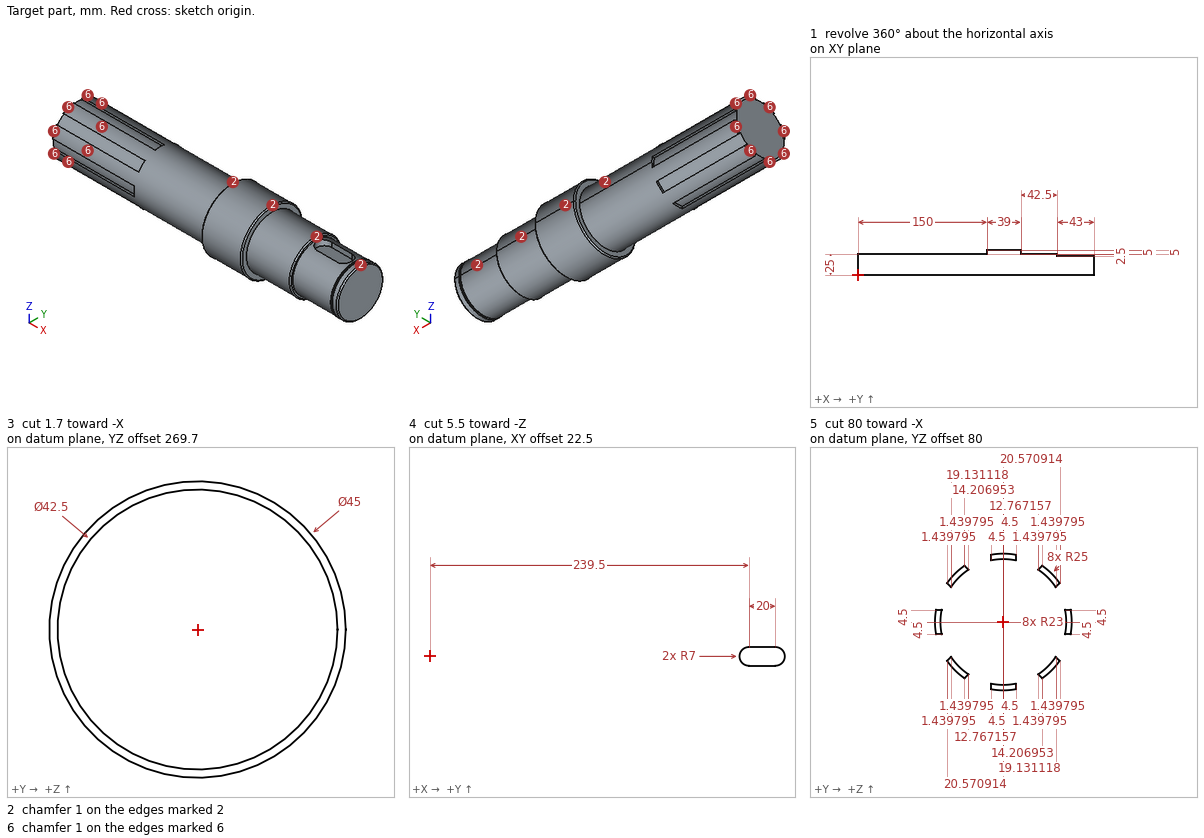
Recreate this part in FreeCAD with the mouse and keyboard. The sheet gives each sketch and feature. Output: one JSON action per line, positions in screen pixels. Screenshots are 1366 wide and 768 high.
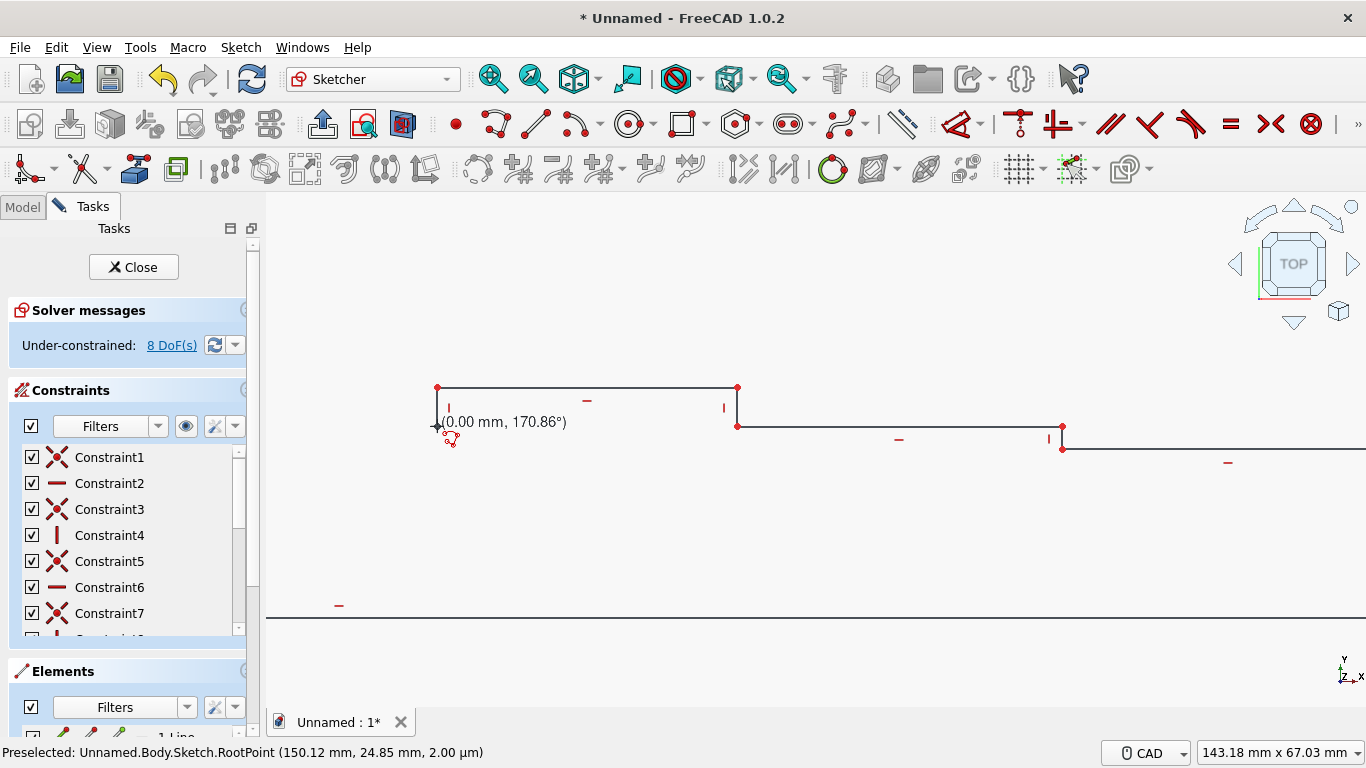
{"action": "scroll", "coordinate": [924, 427], "scroll_direction": "down", "scroll_amount": 6}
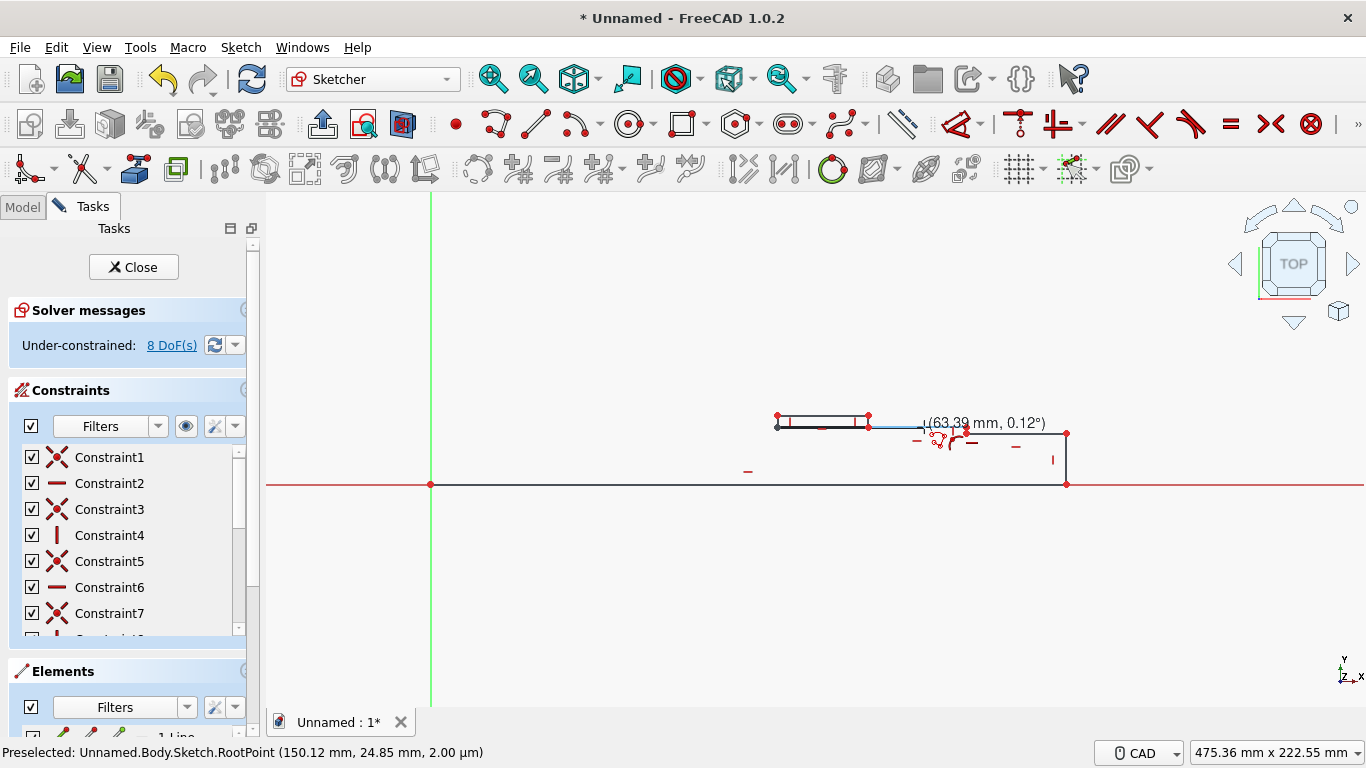
{"action": "left_click", "coordinate": [440, 427]}
{"action": "left_click", "coordinate": [431, 485]}
{"action": "key", "text": "Escape"}
{"action": "key", "text": "Escape"}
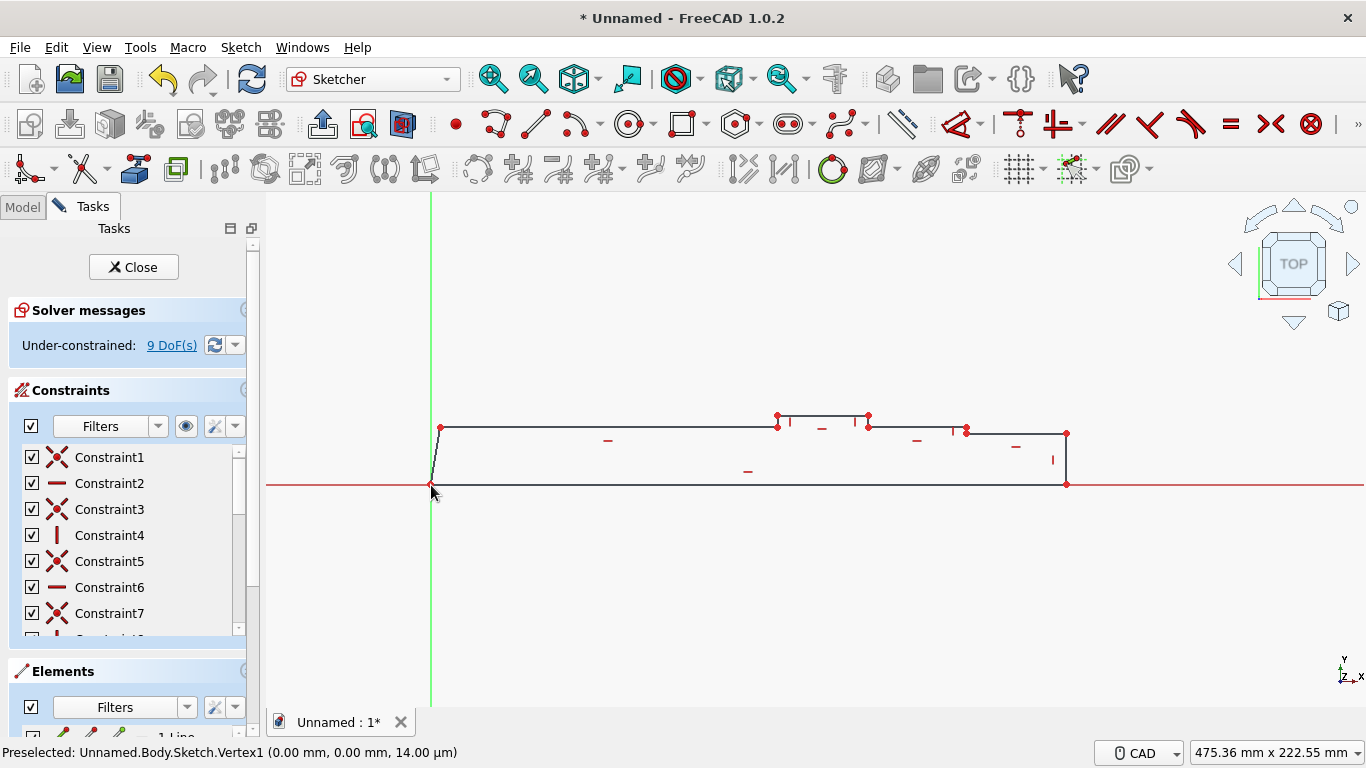
{"action": "left_click", "coordinate": [433, 468]}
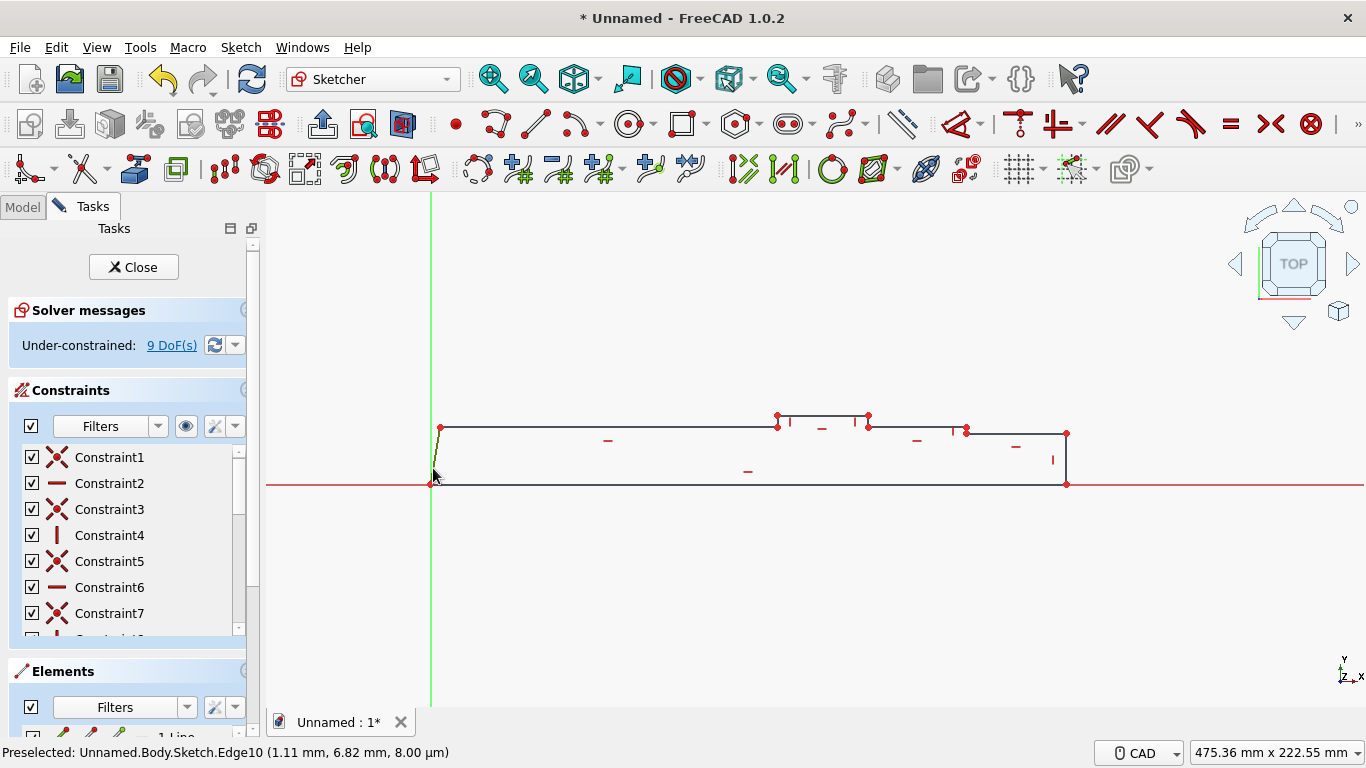
{"action": "key", "text": "v"}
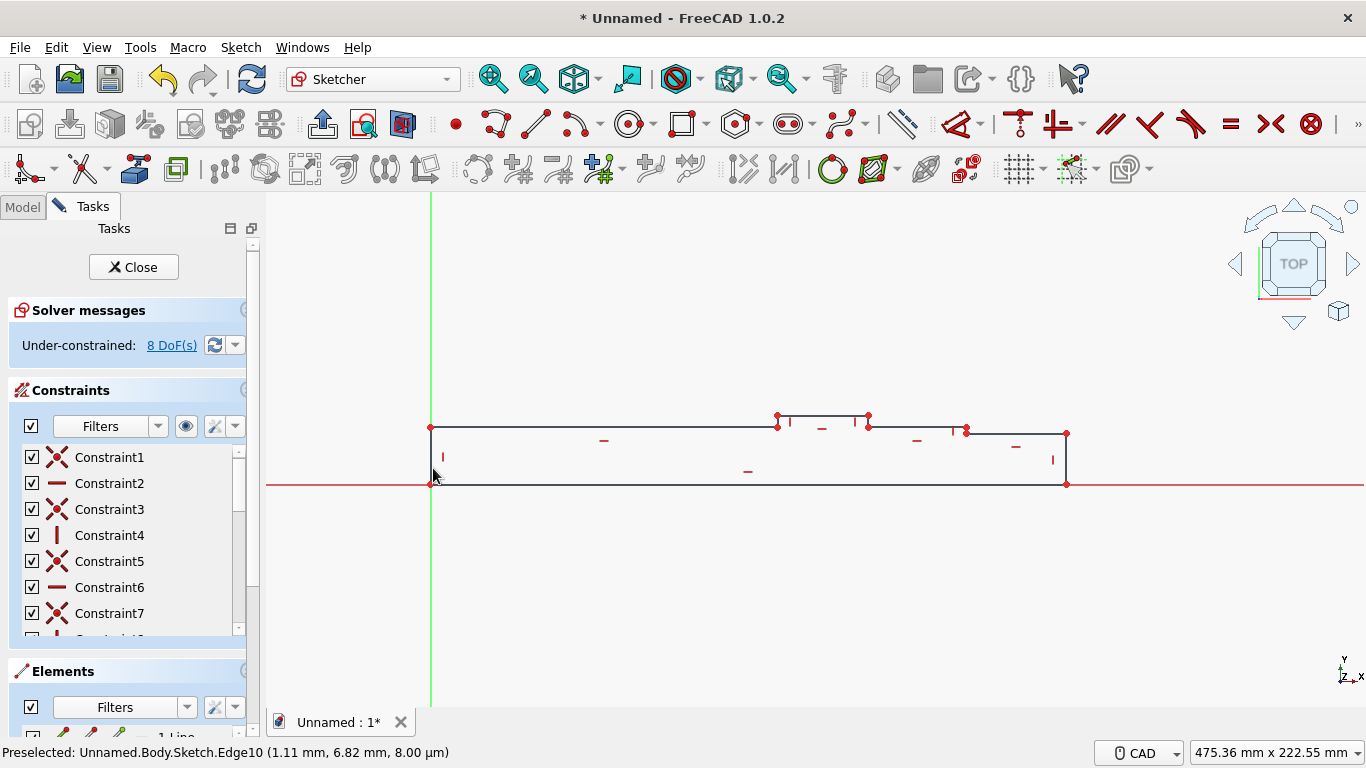
{"action": "scroll", "coordinate": [868, 421], "scroll_direction": "up", "scroll_amount": 7}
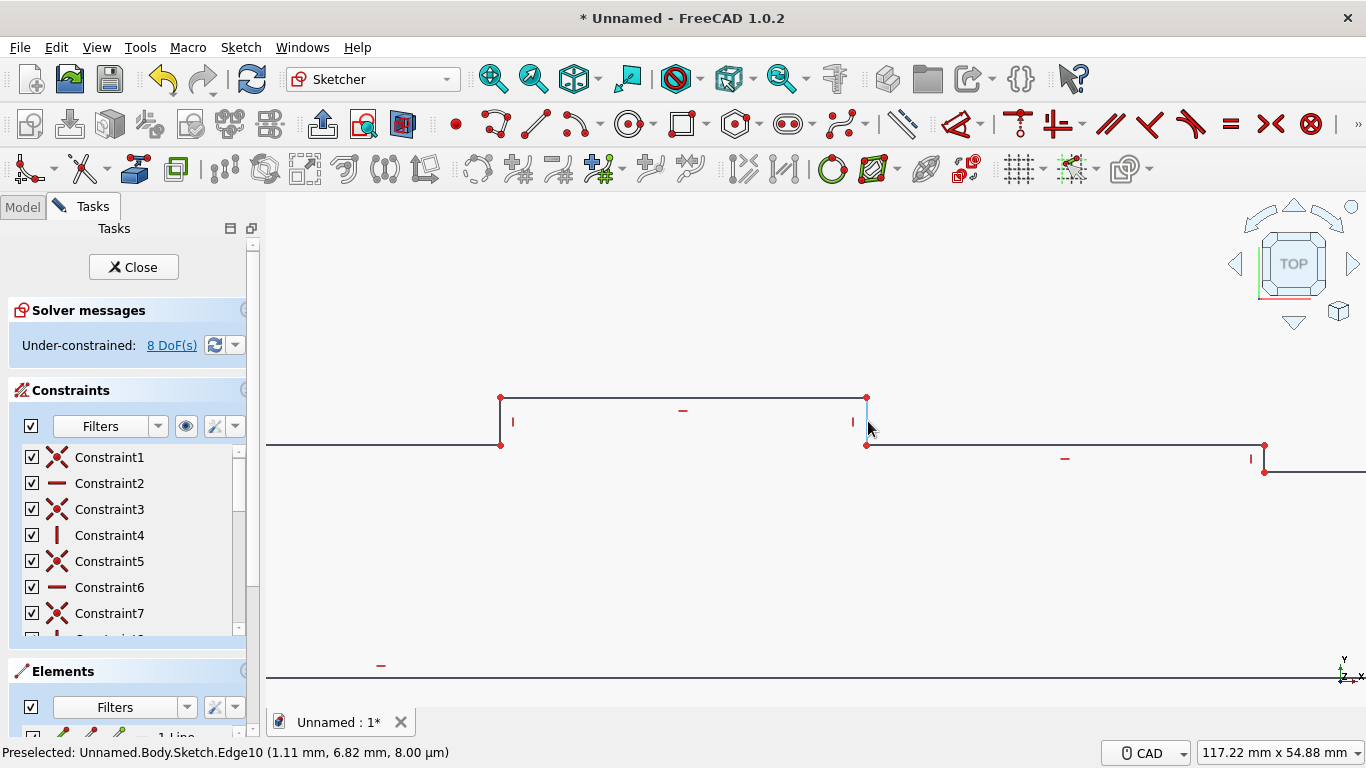
{"action": "left_click", "coordinate": [867, 421]}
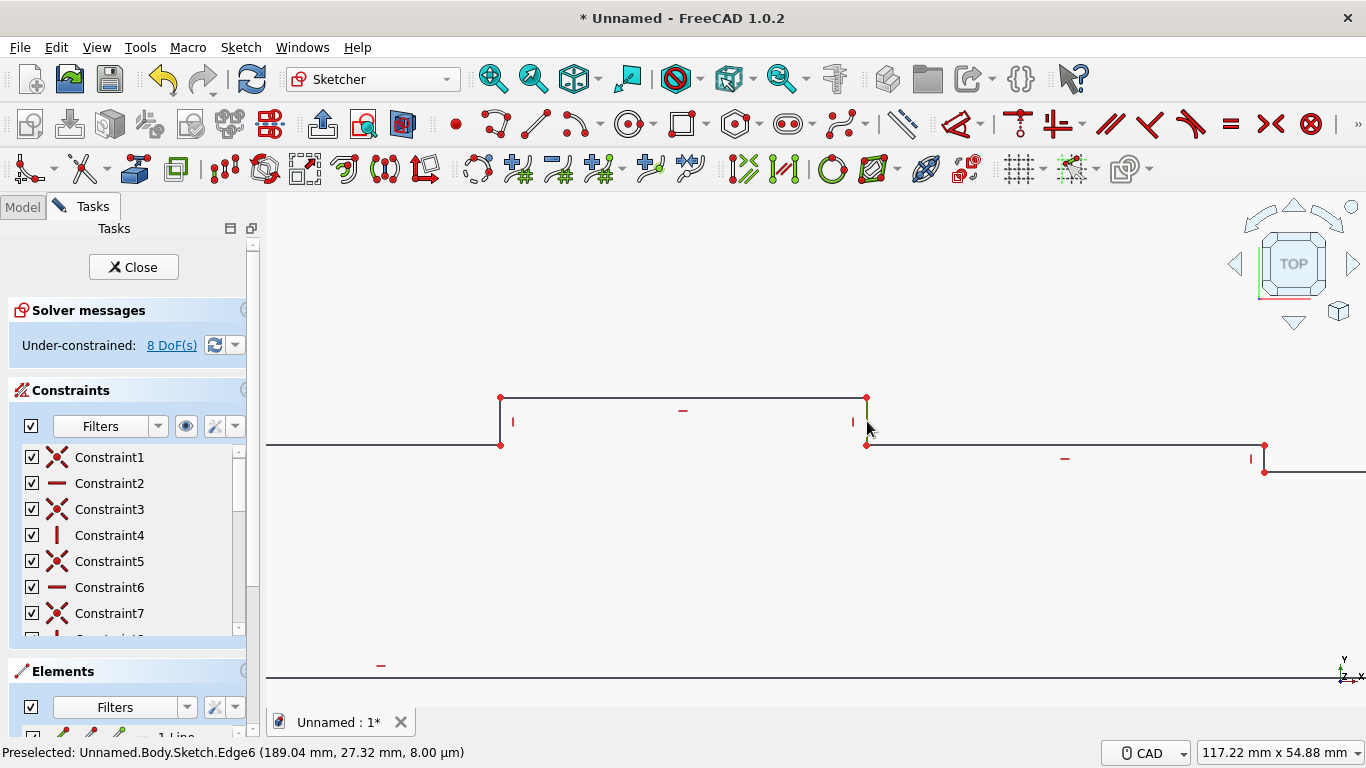
{"action": "key", "text": "i"}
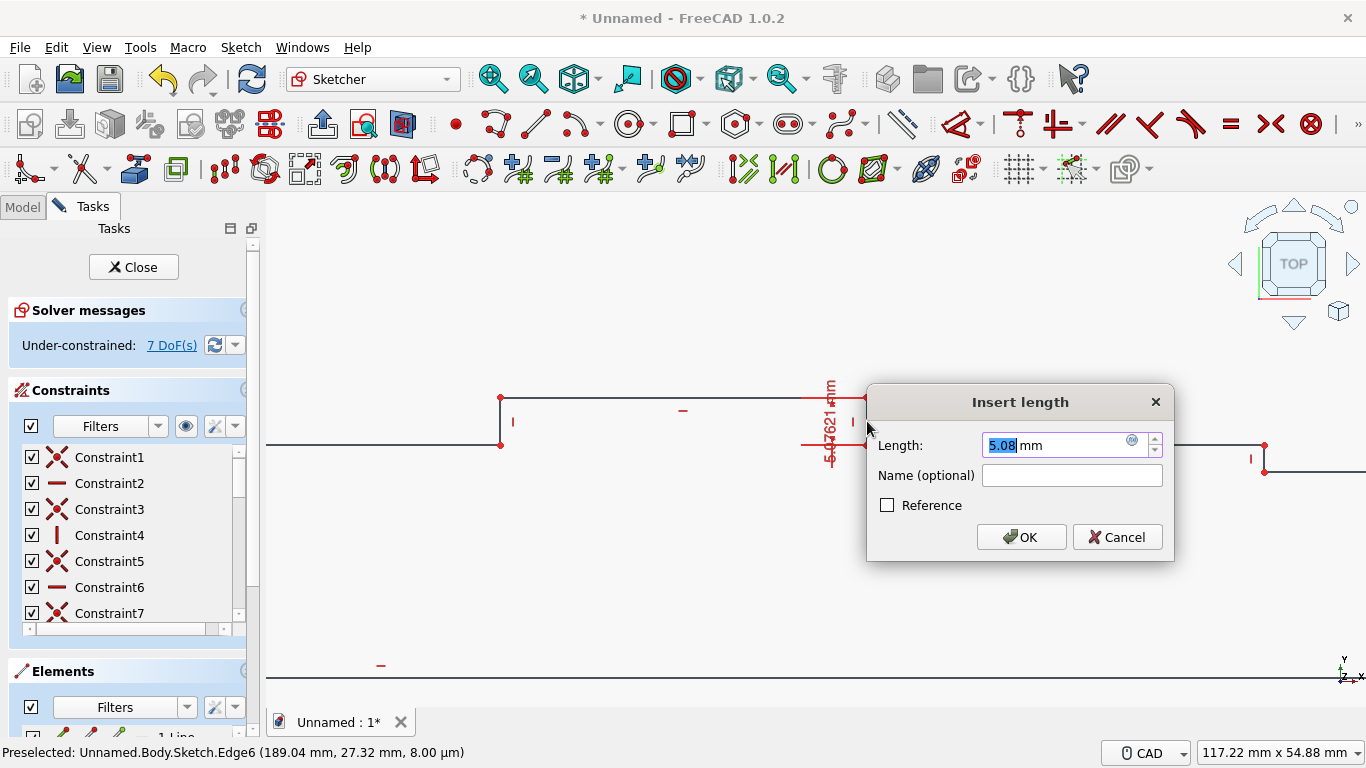
{"action": "type", "text": "5"}
{"action": "key", "text": "Return"}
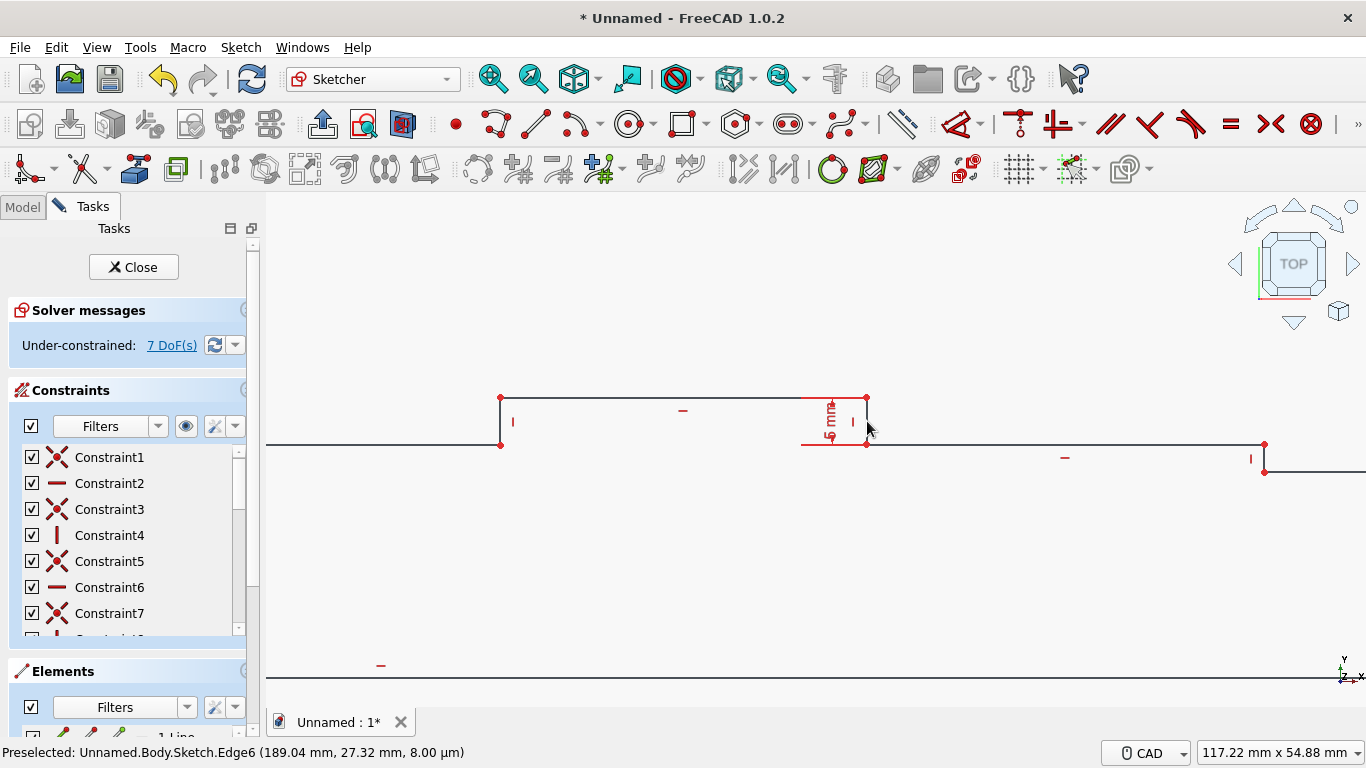
{"action": "left_click", "coordinate": [500, 412]}